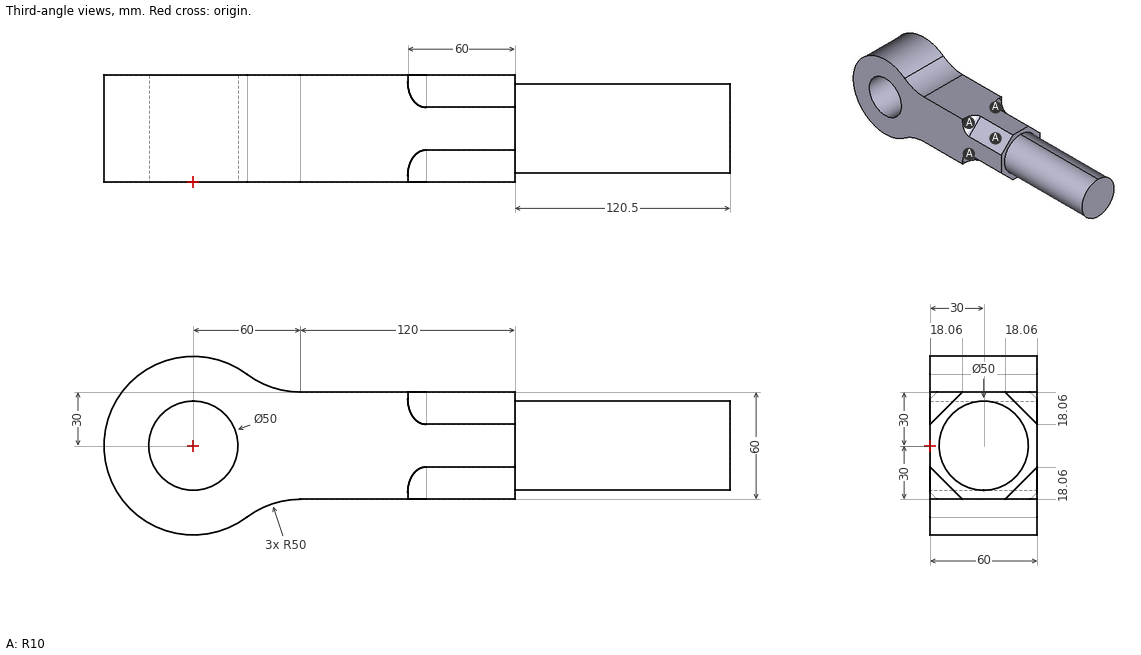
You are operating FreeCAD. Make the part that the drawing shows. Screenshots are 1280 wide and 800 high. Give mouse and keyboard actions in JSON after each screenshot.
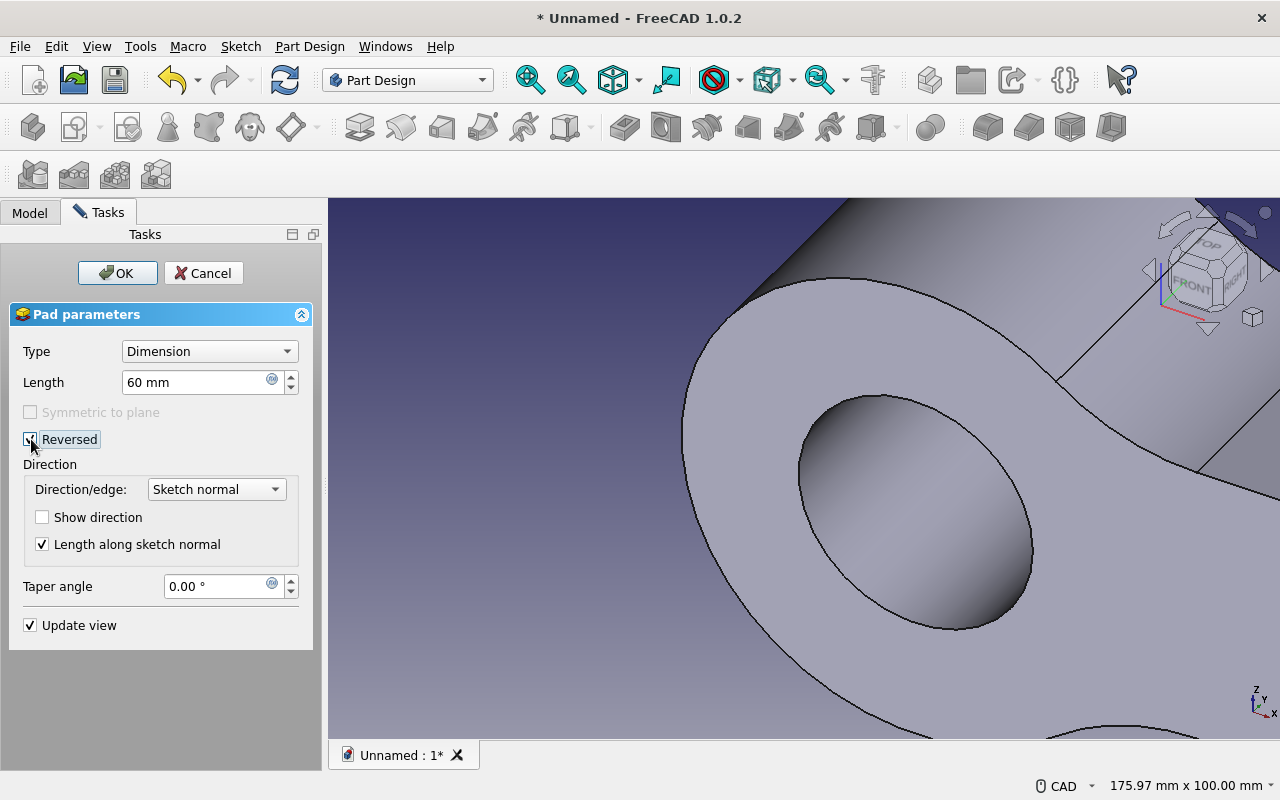
{"action": "left_click", "coordinate": [118, 273]}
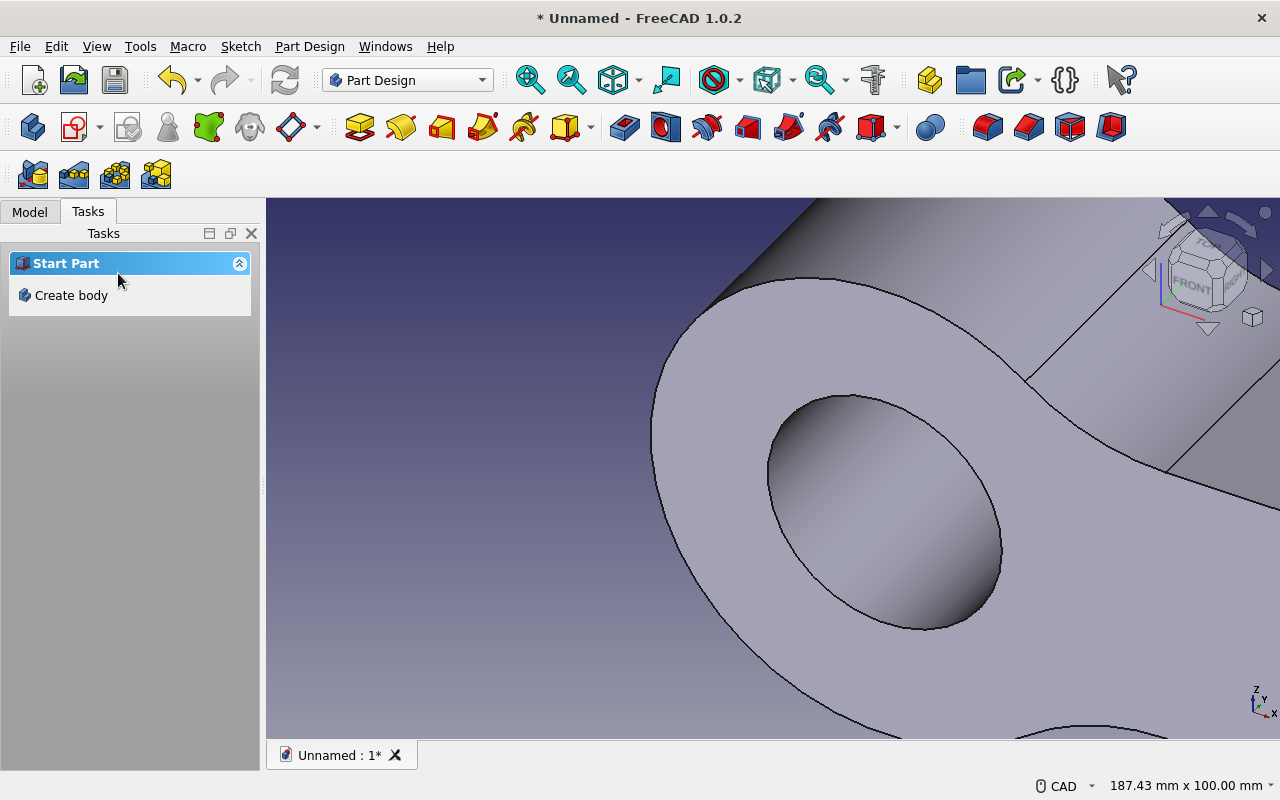
{"action": "key", "text": "v f"}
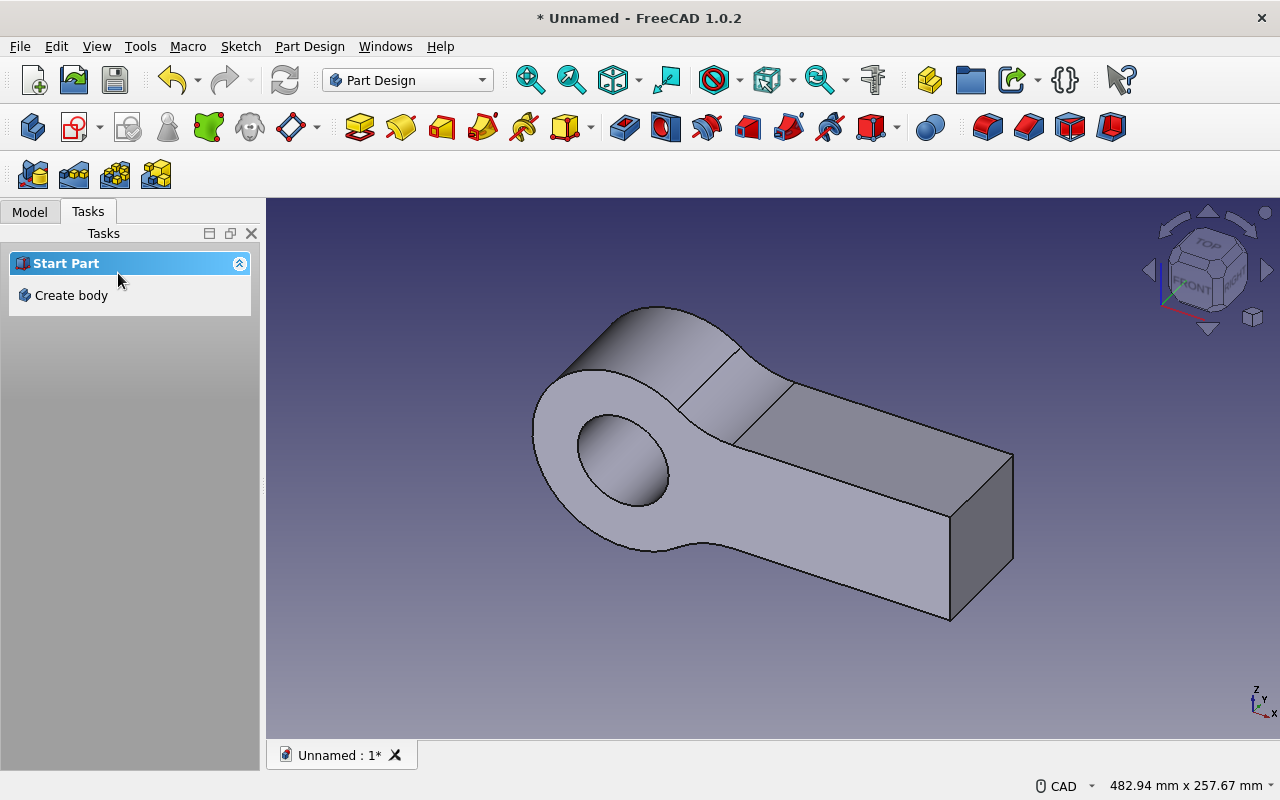
{"action": "left_click", "coordinate": [982, 537]}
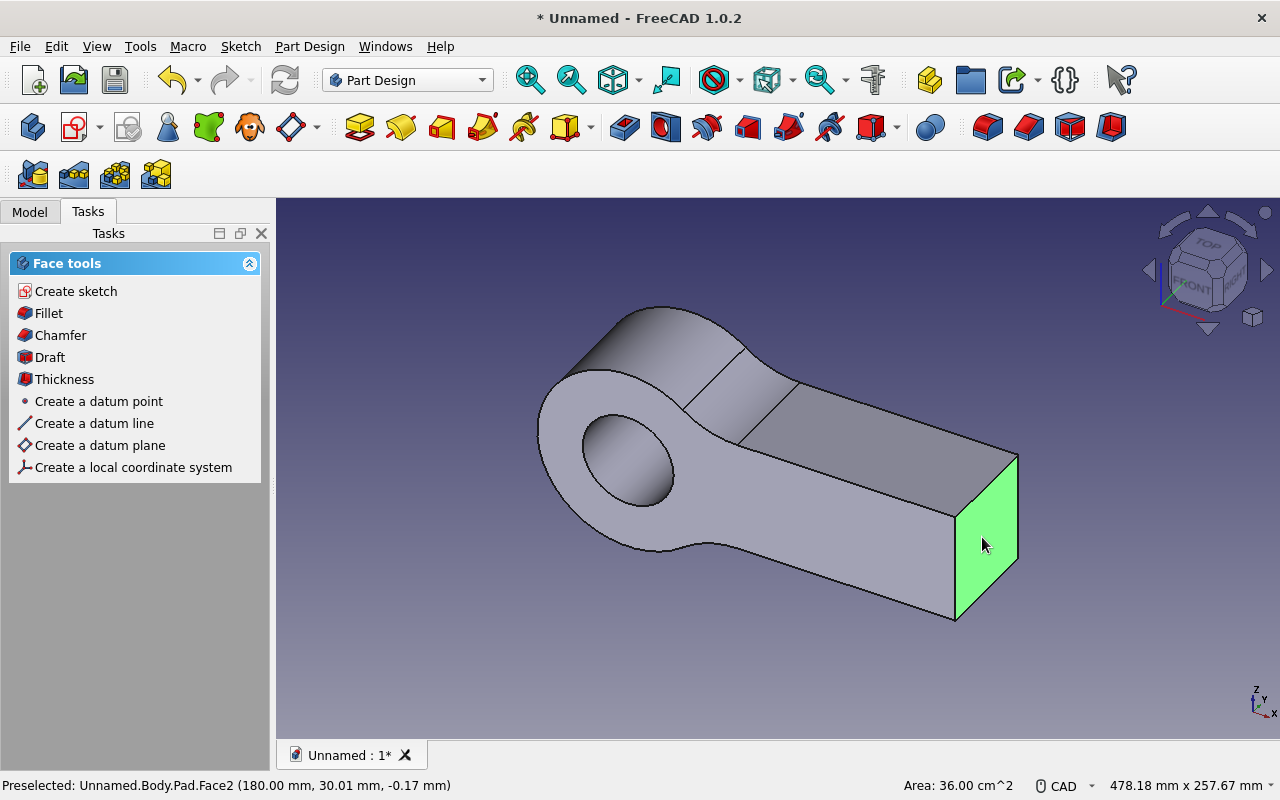
{"action": "left_click", "coordinate": [74, 128]}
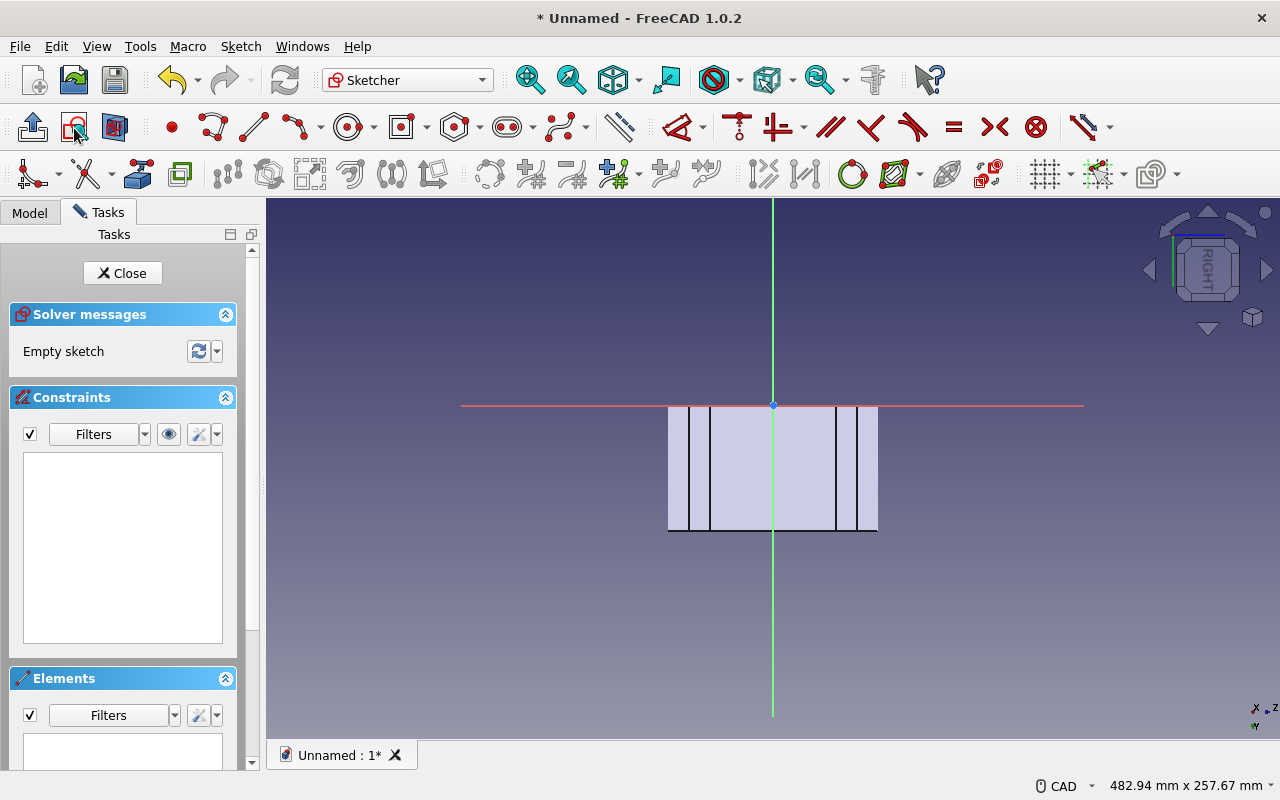
{"action": "scroll", "coordinate": [813, 468], "scroll_direction": "up", "scroll_amount": 5}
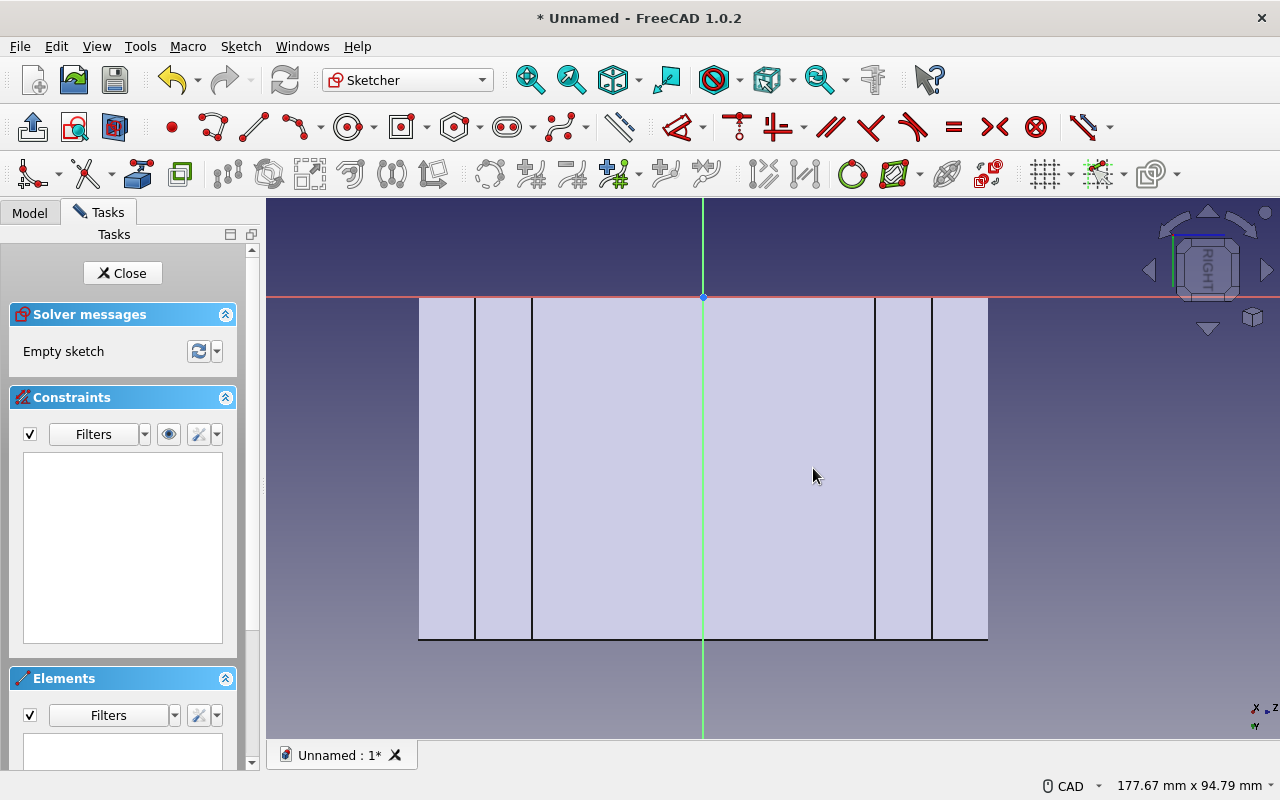
{"action": "key", "text": "g m"}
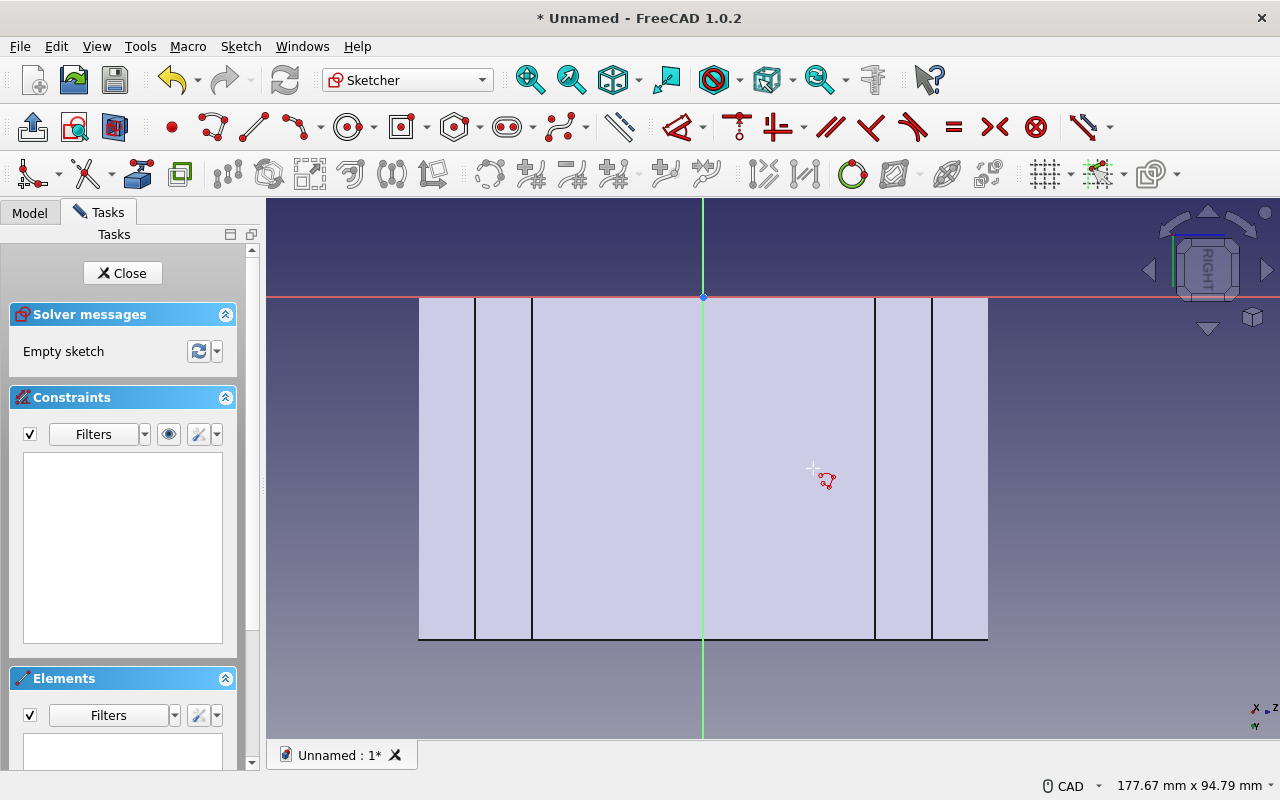
{"action": "left_click", "coordinate": [875, 537]}
{"action": "left_click", "coordinate": [771, 640]}
{"action": "left_click", "coordinate": [875, 640]}
{"action": "left_click", "coordinate": [875, 538]}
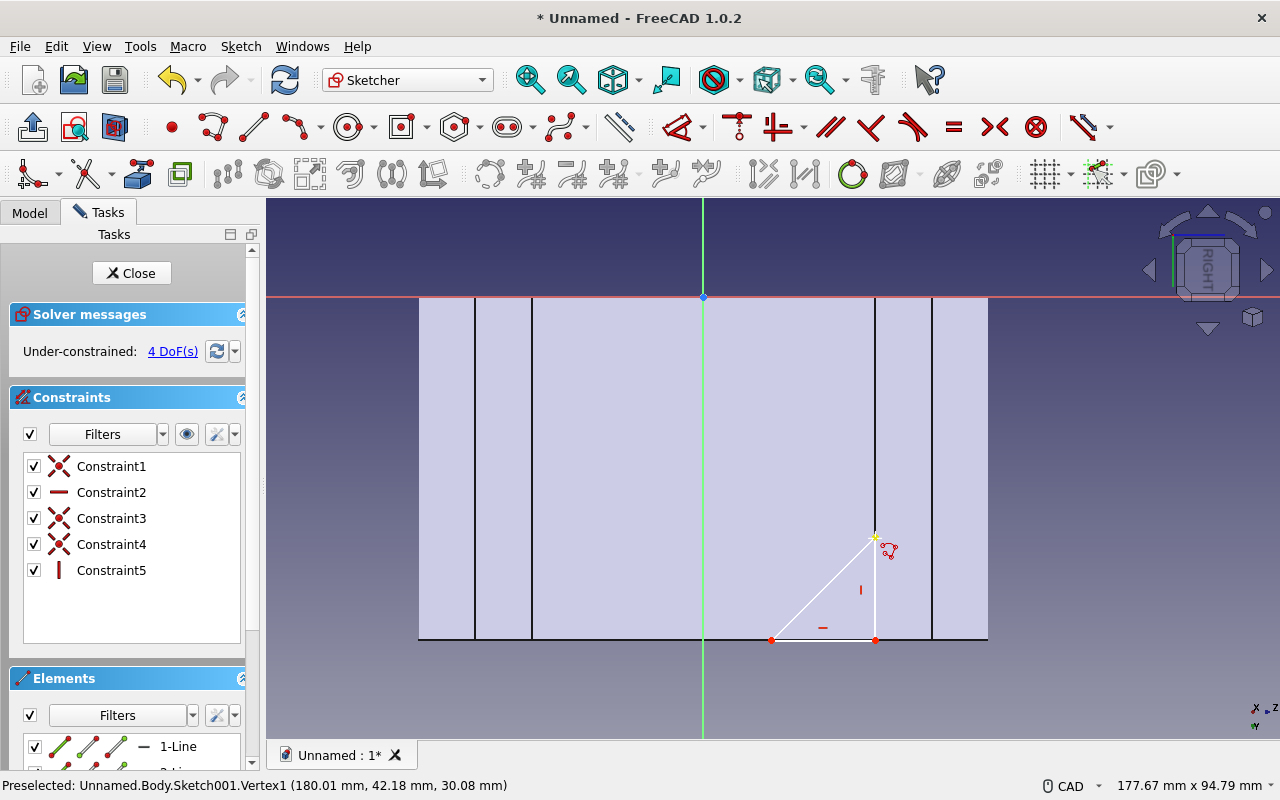
{"action": "left_click", "coordinate": [532, 537]}
{"action": "left_click", "coordinate": [532, 640]}
{"action": "left_click", "coordinate": [635, 640]}
{"action": "left_click", "coordinate": [532, 538]}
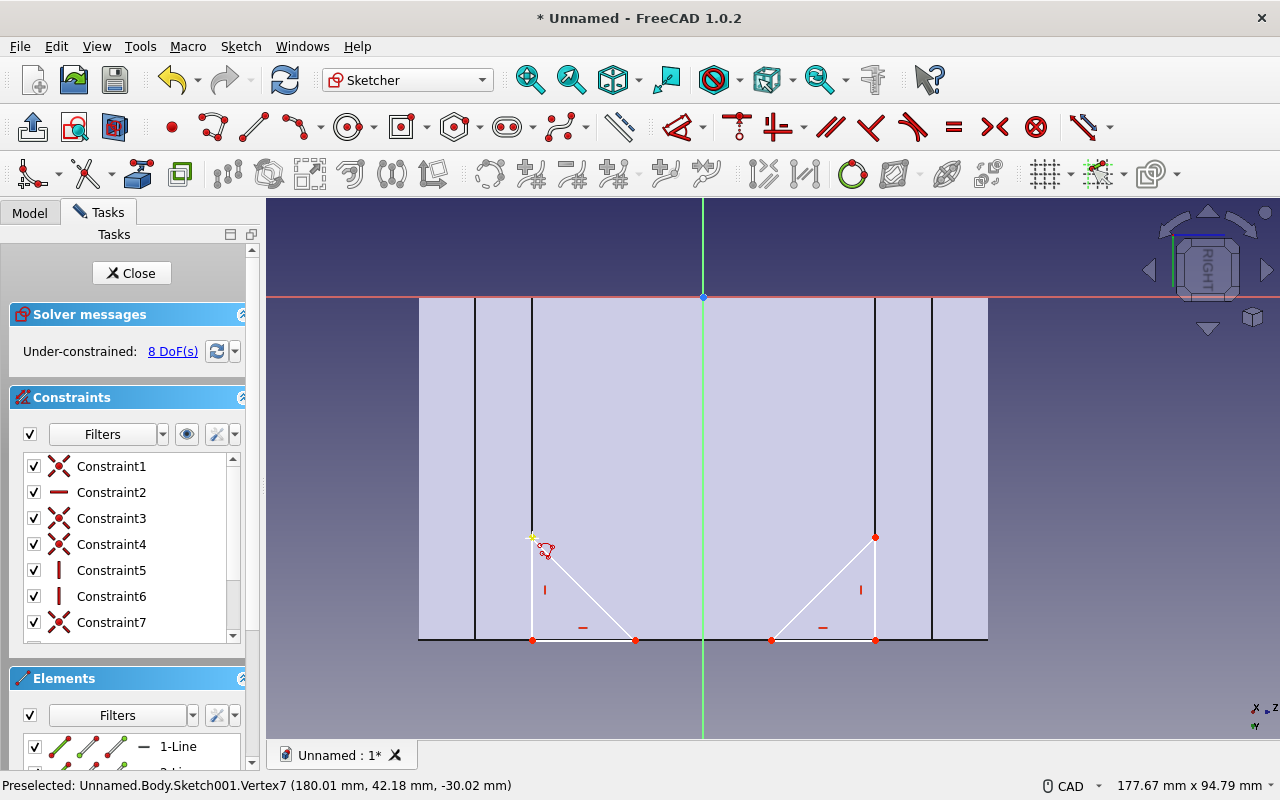
{"action": "left_click", "coordinate": [771, 297]}
{"action": "left_click", "coordinate": [875, 400]}
{"action": "left_click", "coordinate": [875, 306]}
{"action": "left_click", "coordinate": [771, 297]}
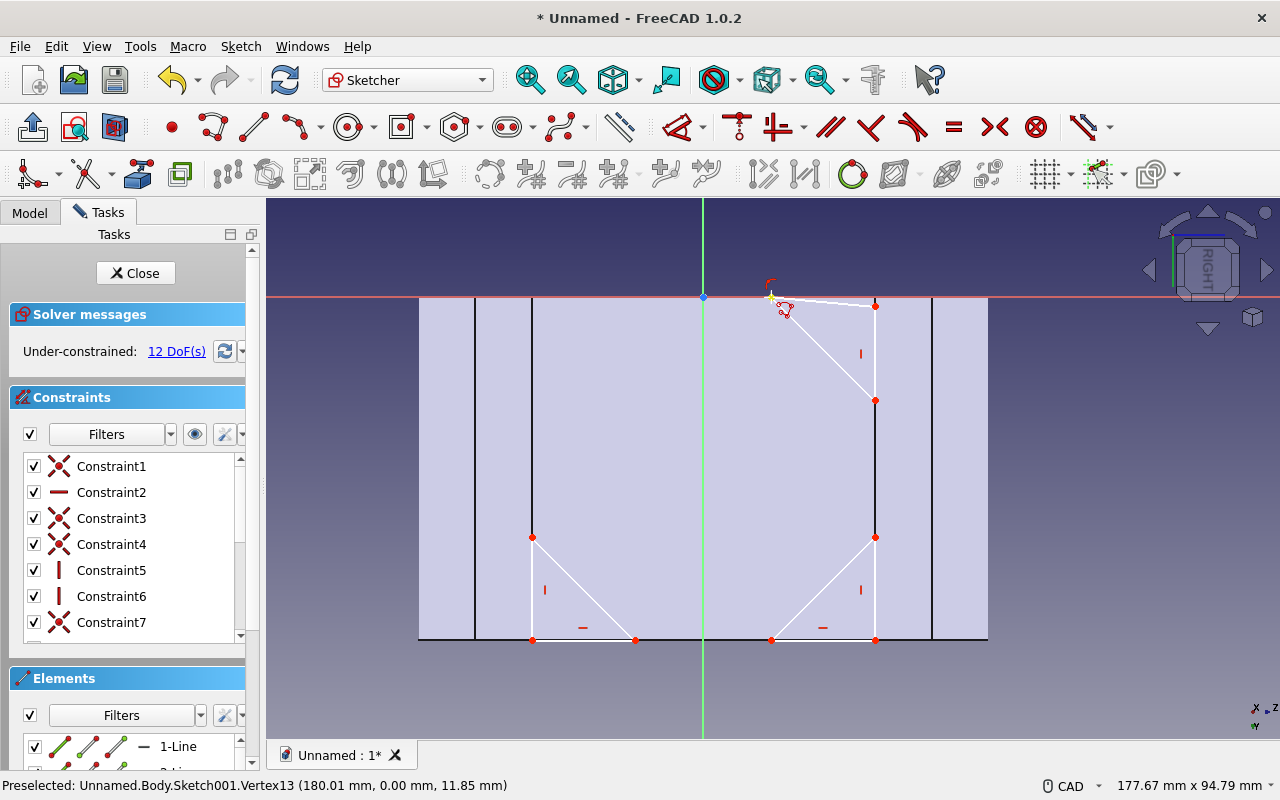
{"action": "left_click", "coordinate": [635, 297]}
{"action": "left_click", "coordinate": [532, 306]}
{"action": "left_click", "coordinate": [532, 400]}
{"action": "left_click", "coordinate": [635, 297]}
{"action": "key", "text": "Escape"}
{"action": "key", "text": "Escape"}